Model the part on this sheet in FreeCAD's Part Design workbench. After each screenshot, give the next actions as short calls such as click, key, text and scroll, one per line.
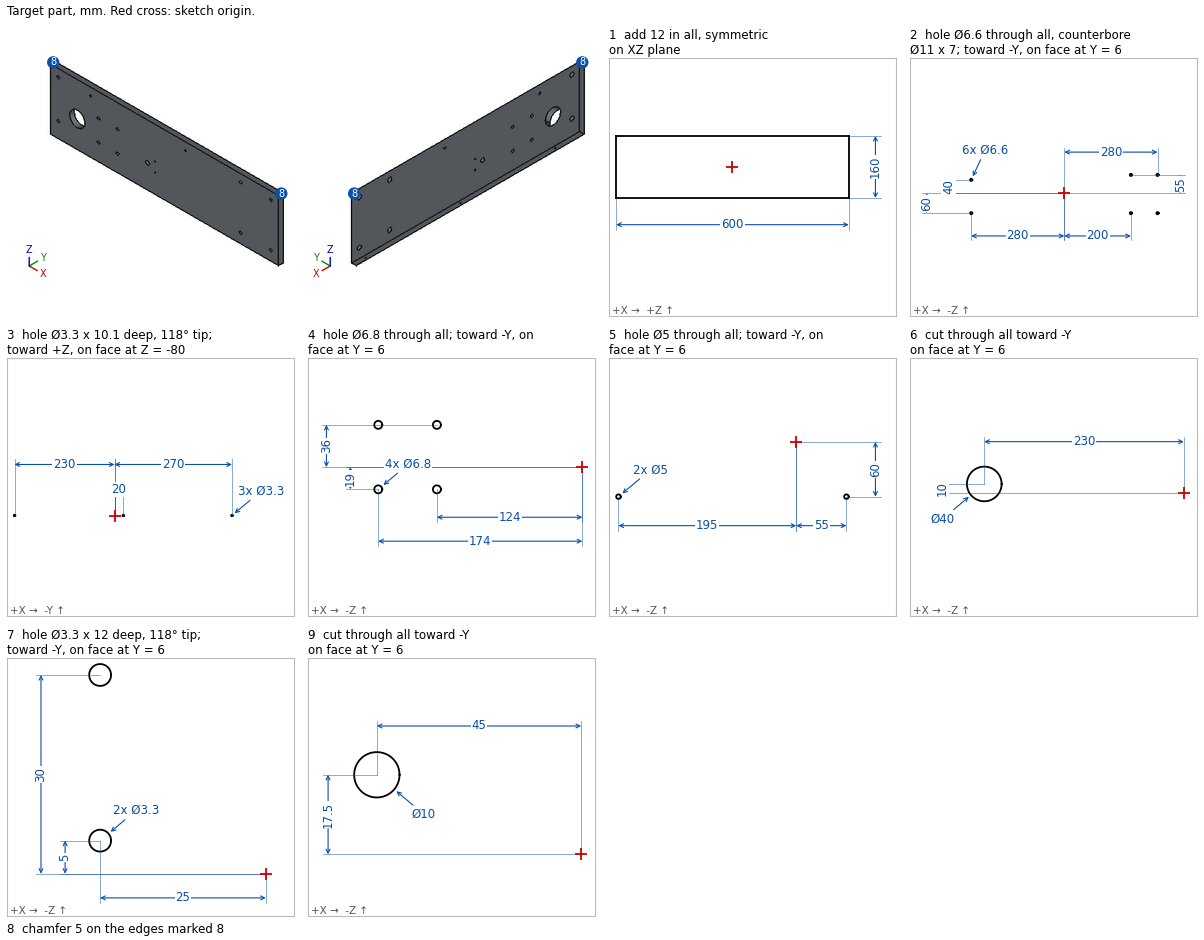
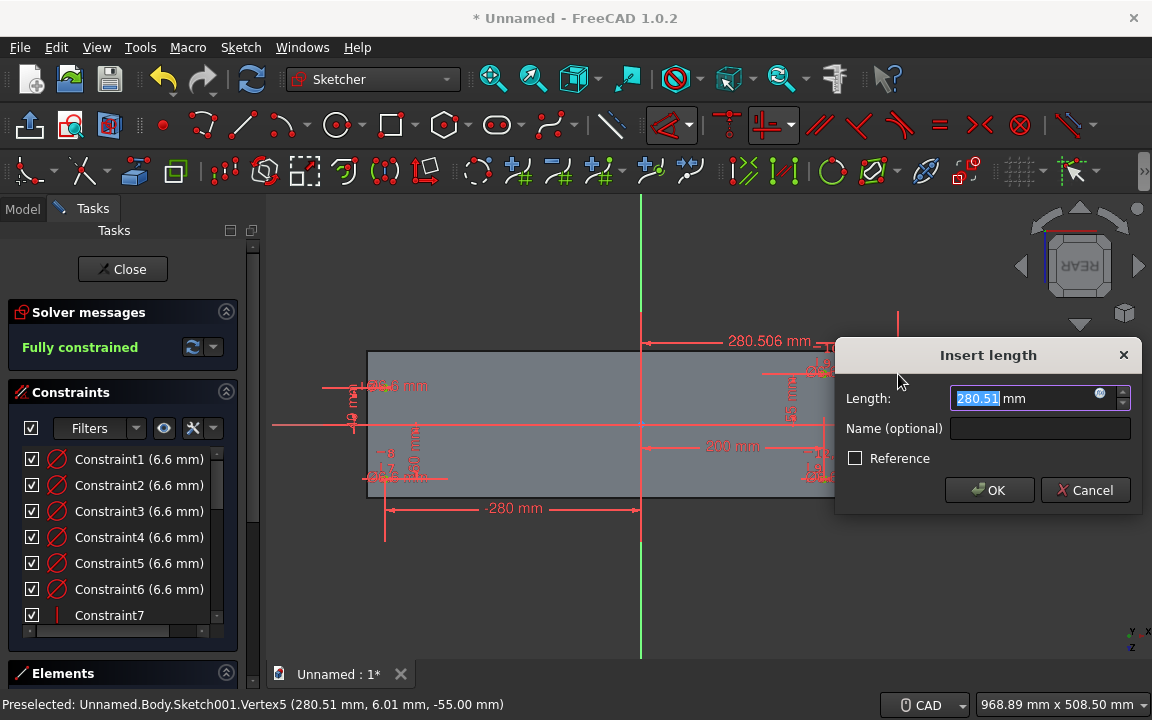
text(280)
key(Return)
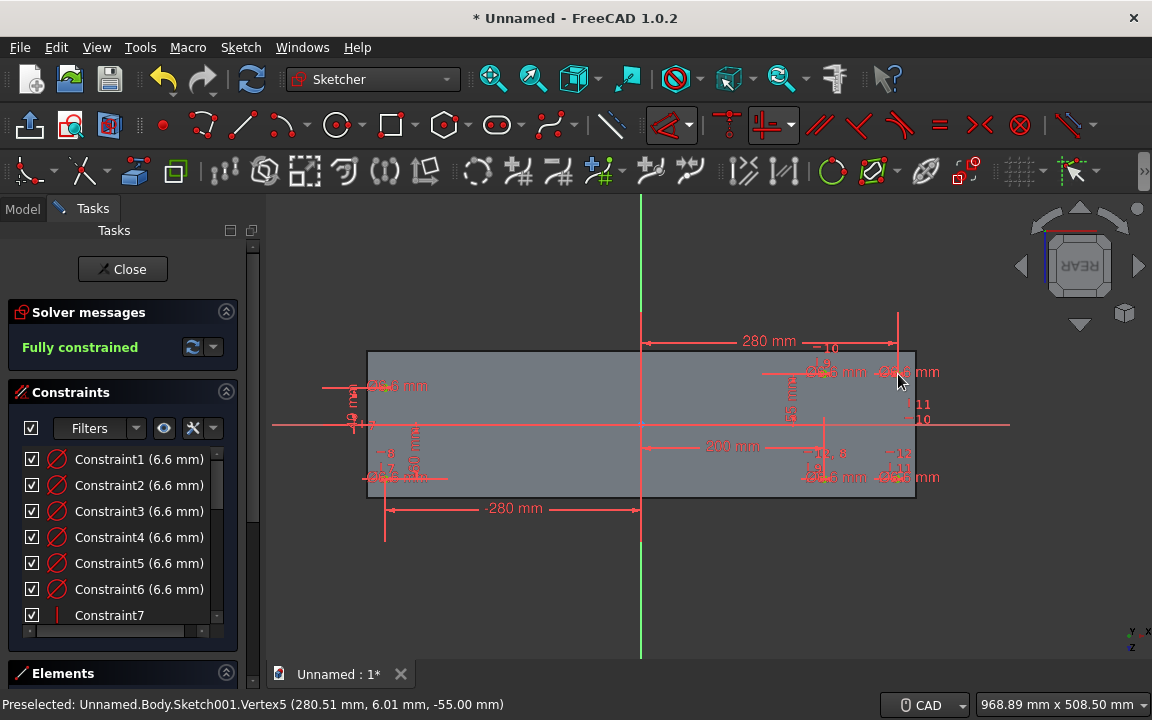
click(123, 269)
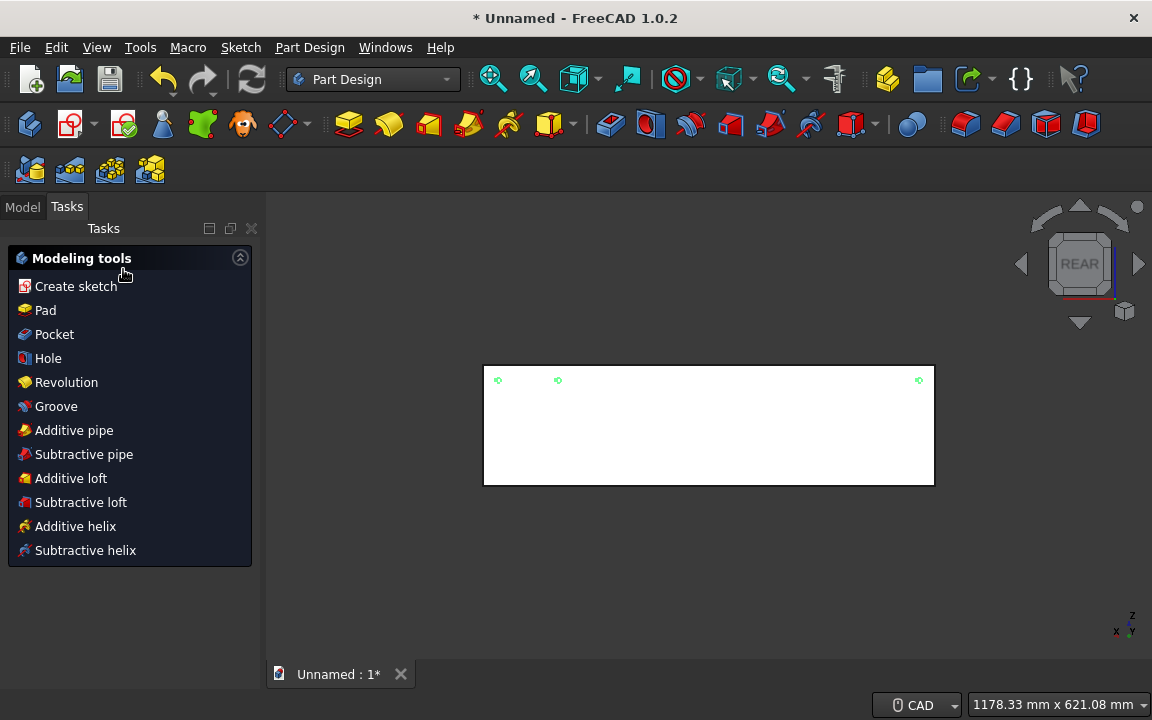
click(652, 124)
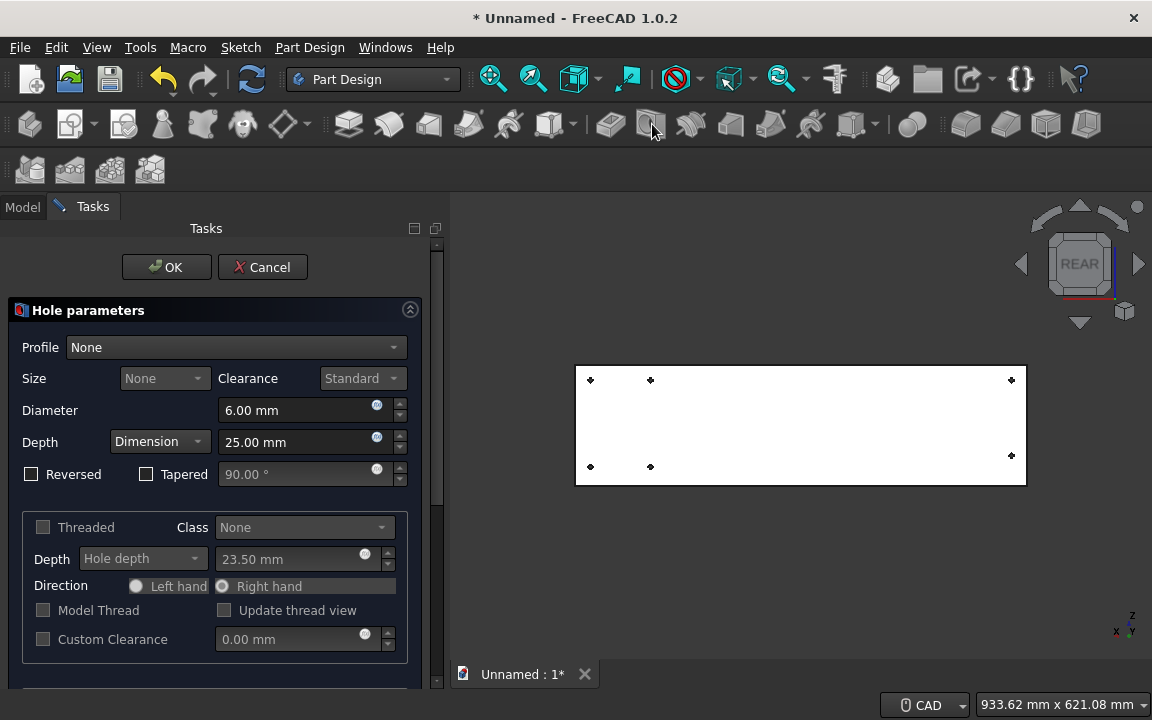
triple_click(305, 410)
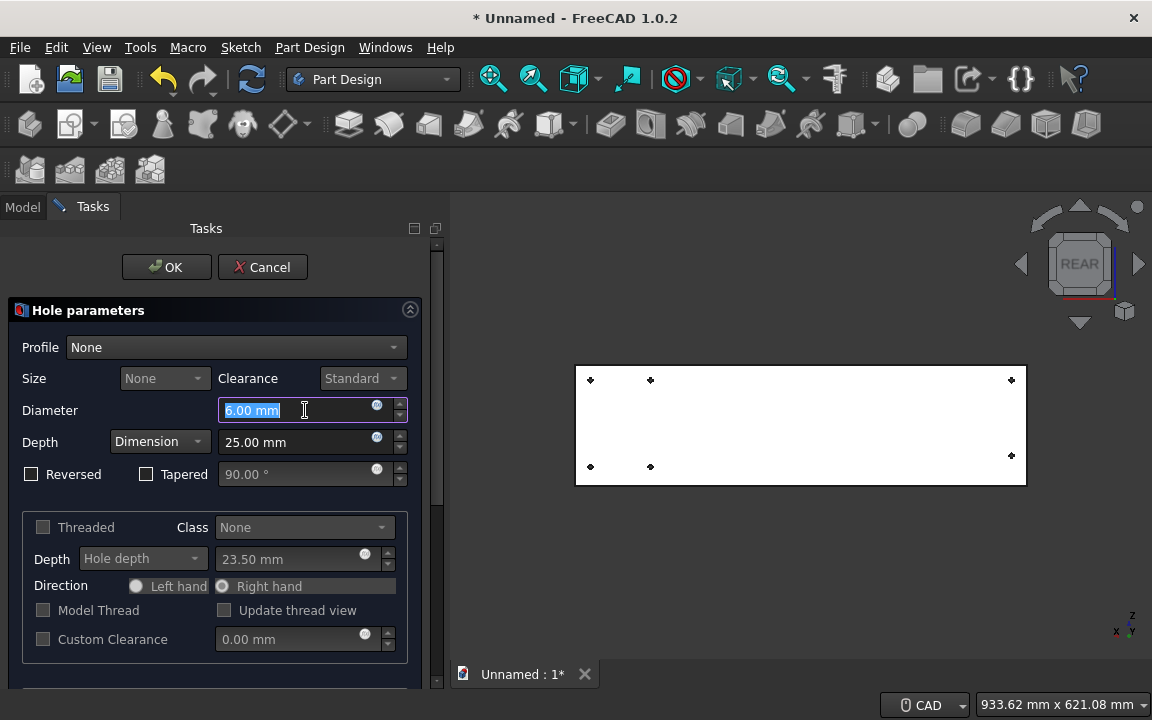
text(6.6)
key(Tab)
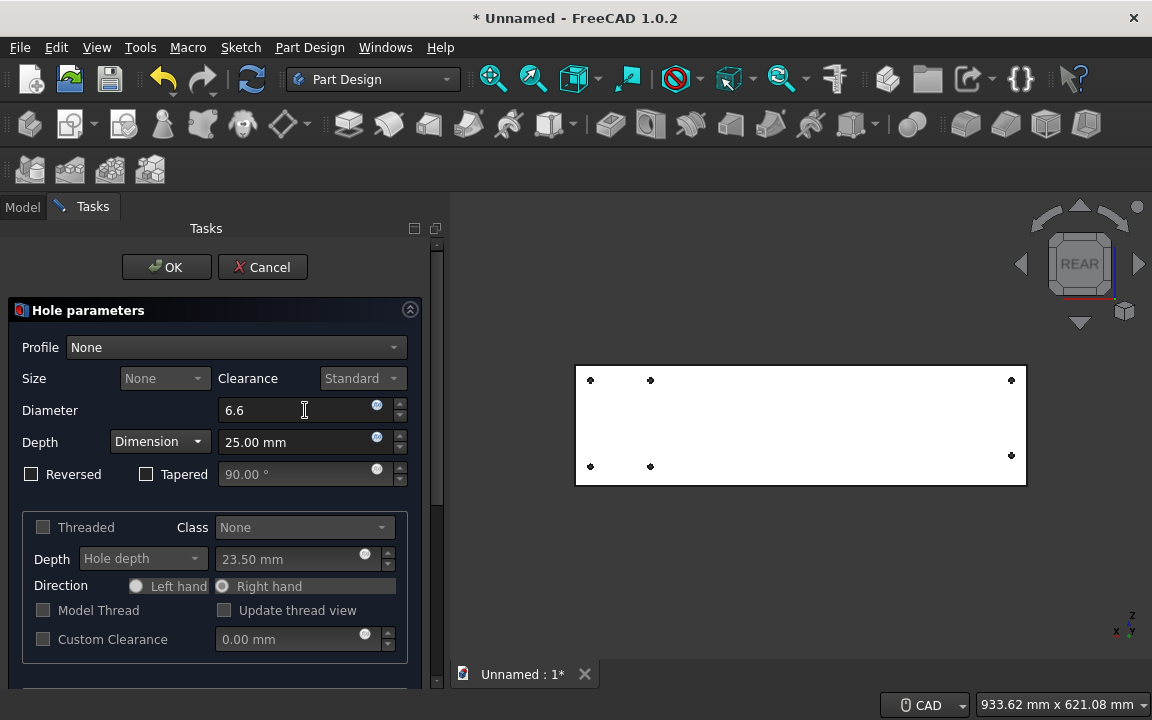
click(161, 442)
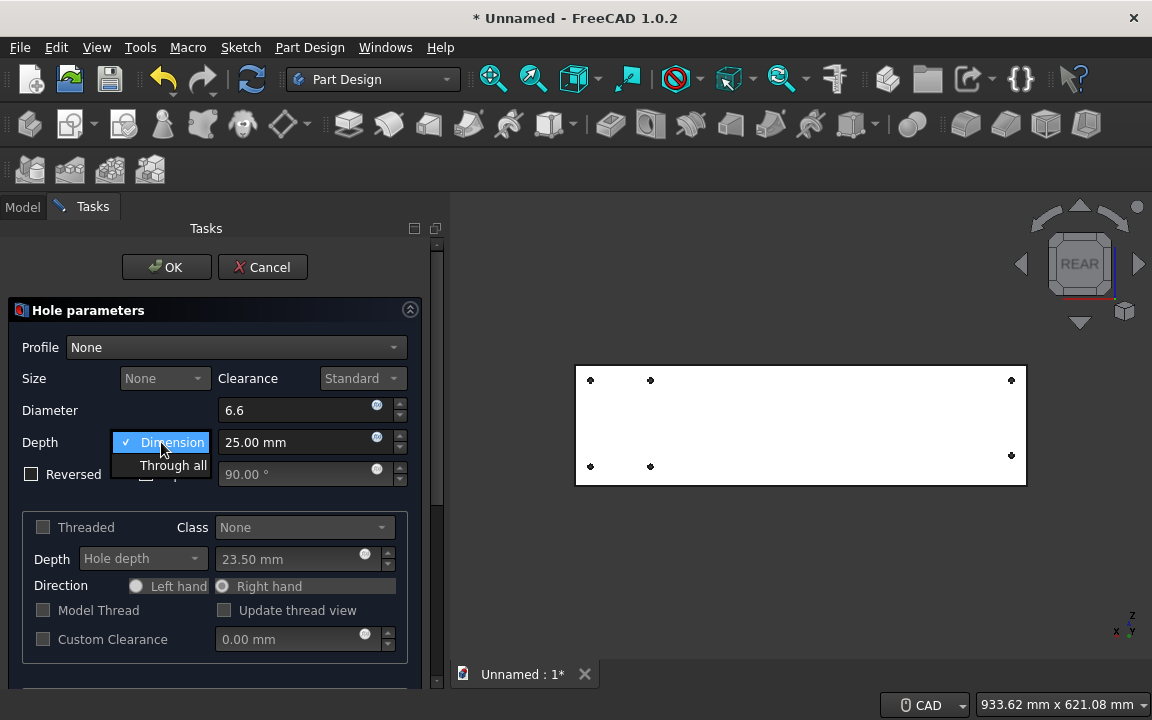
click(160, 466)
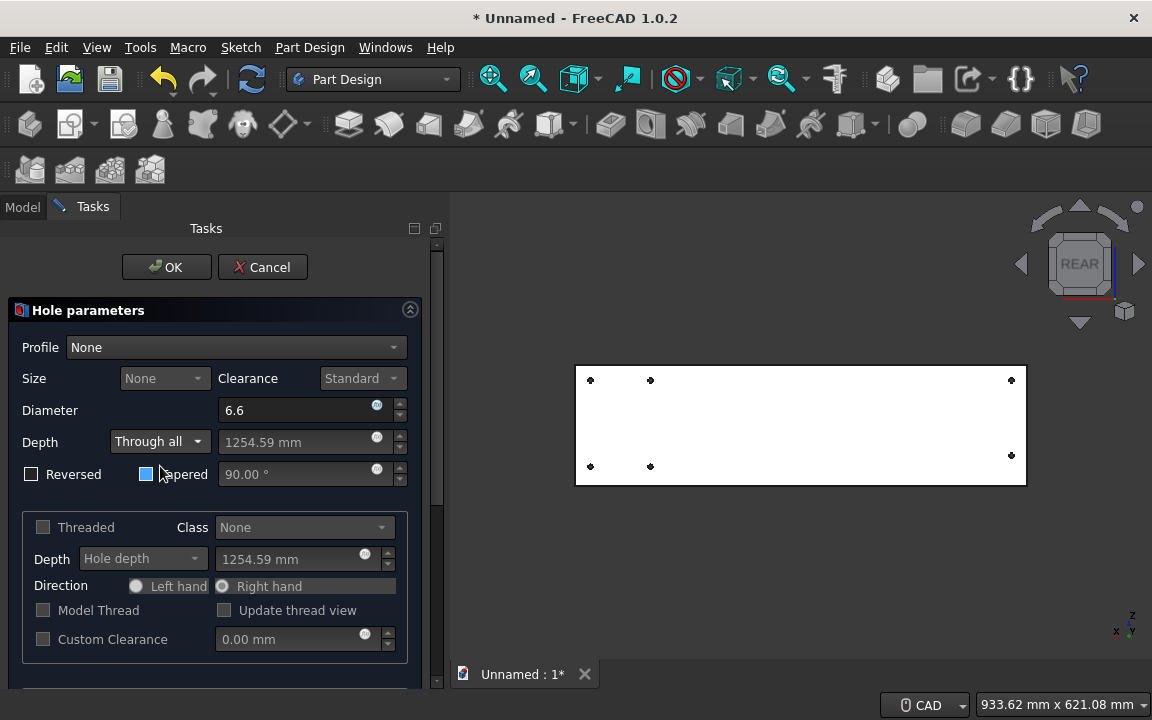
scroll(437, 463, down, 2)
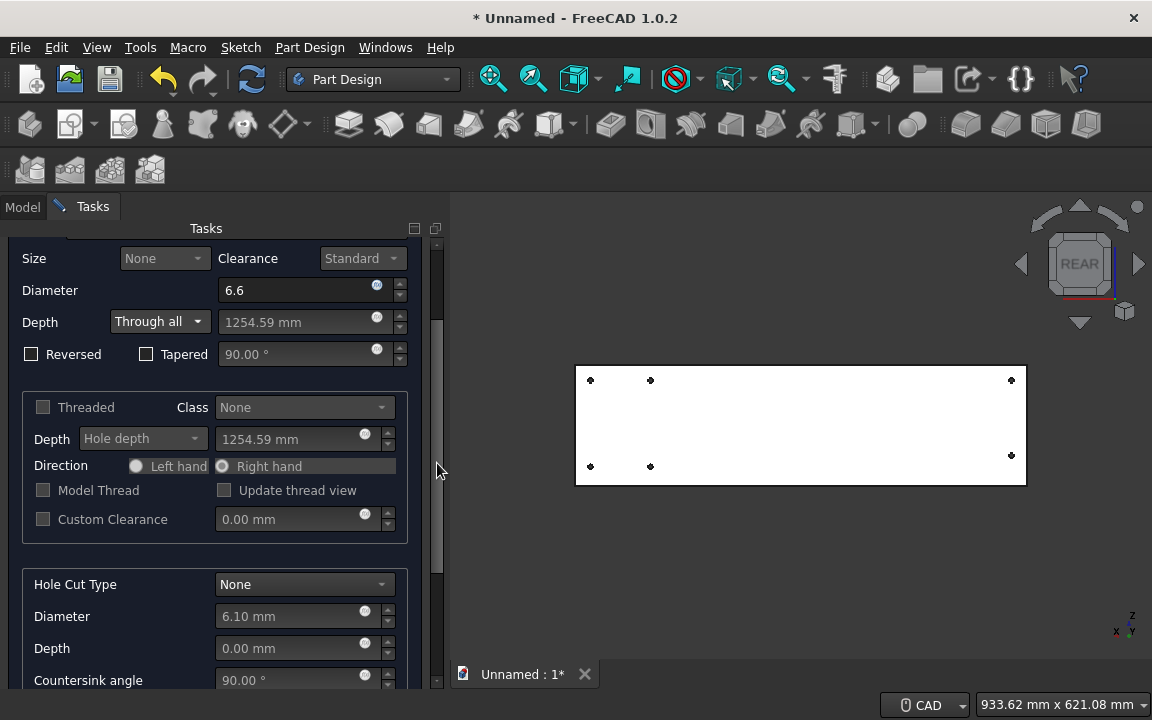
click(306, 584)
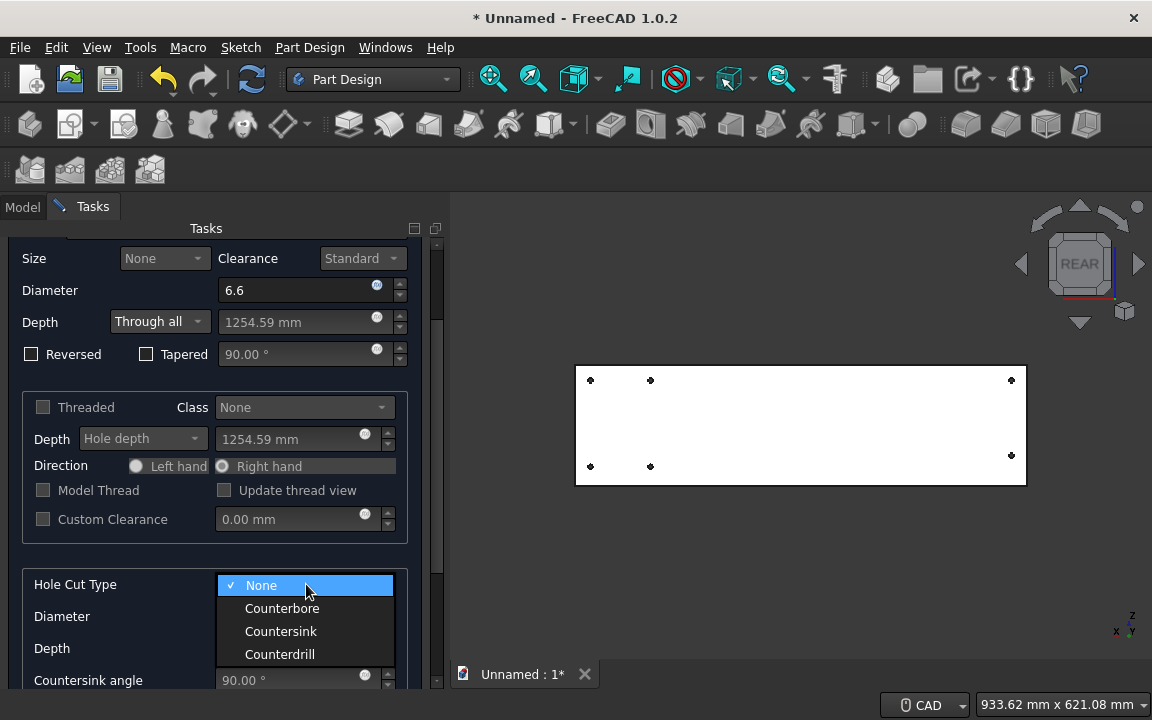
click(304, 608)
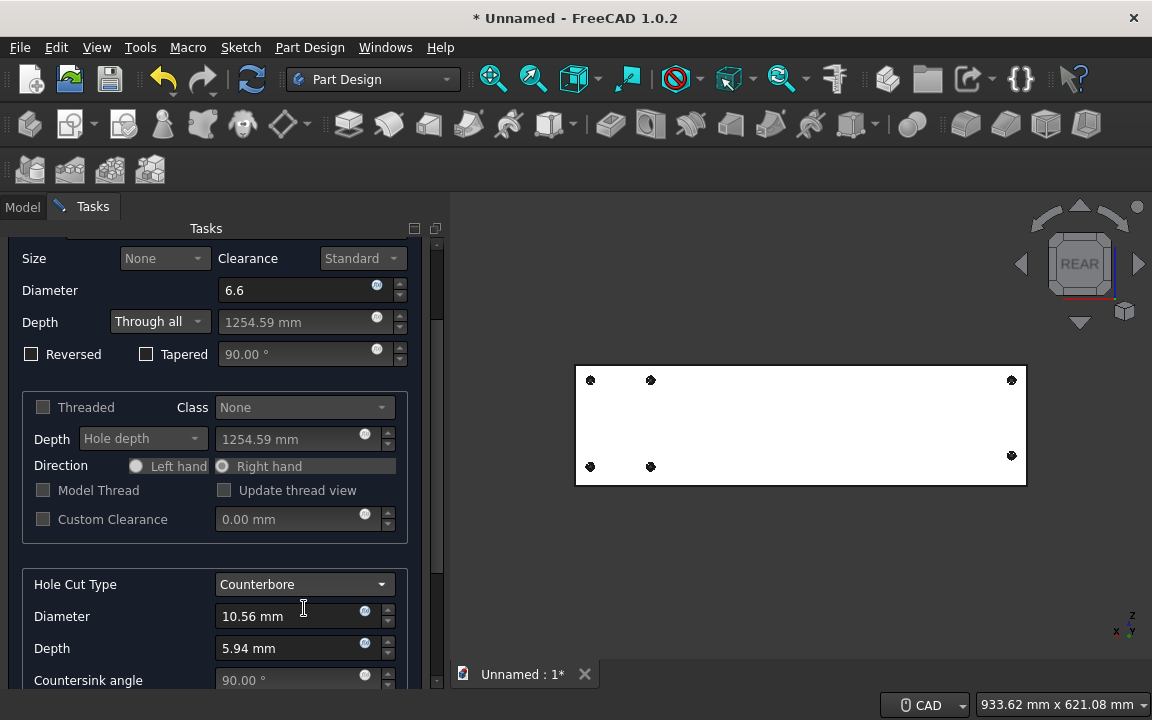
triple_click(298, 616)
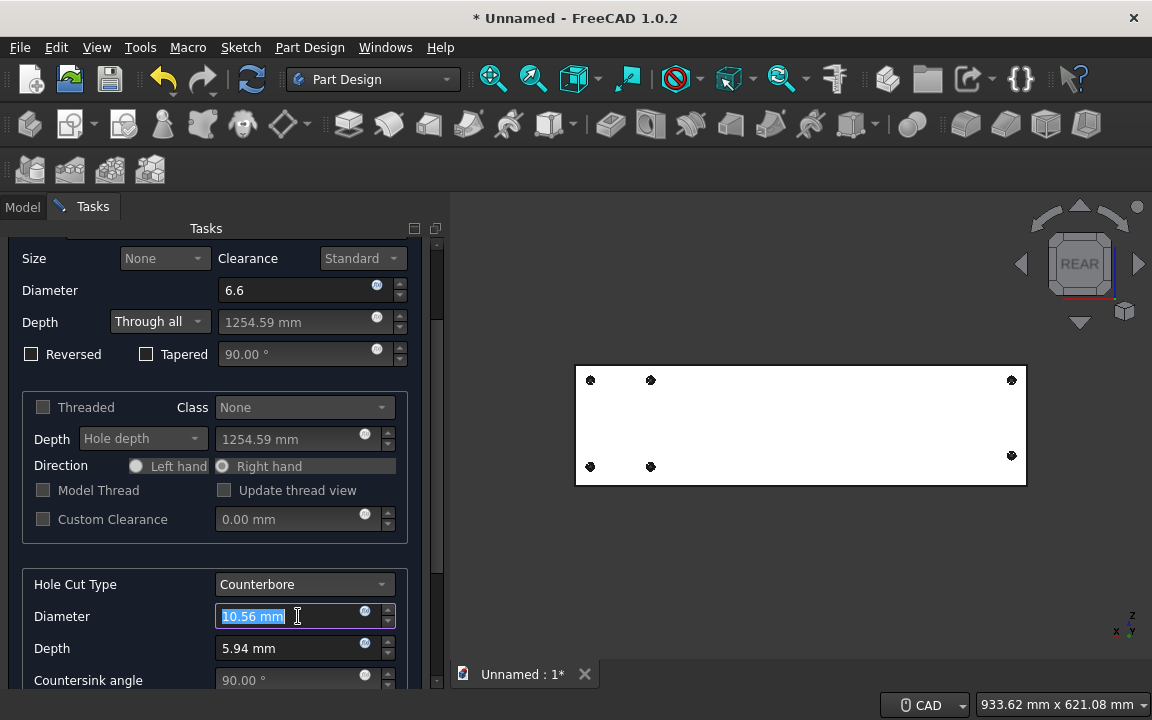
text(11)
key(Tab)